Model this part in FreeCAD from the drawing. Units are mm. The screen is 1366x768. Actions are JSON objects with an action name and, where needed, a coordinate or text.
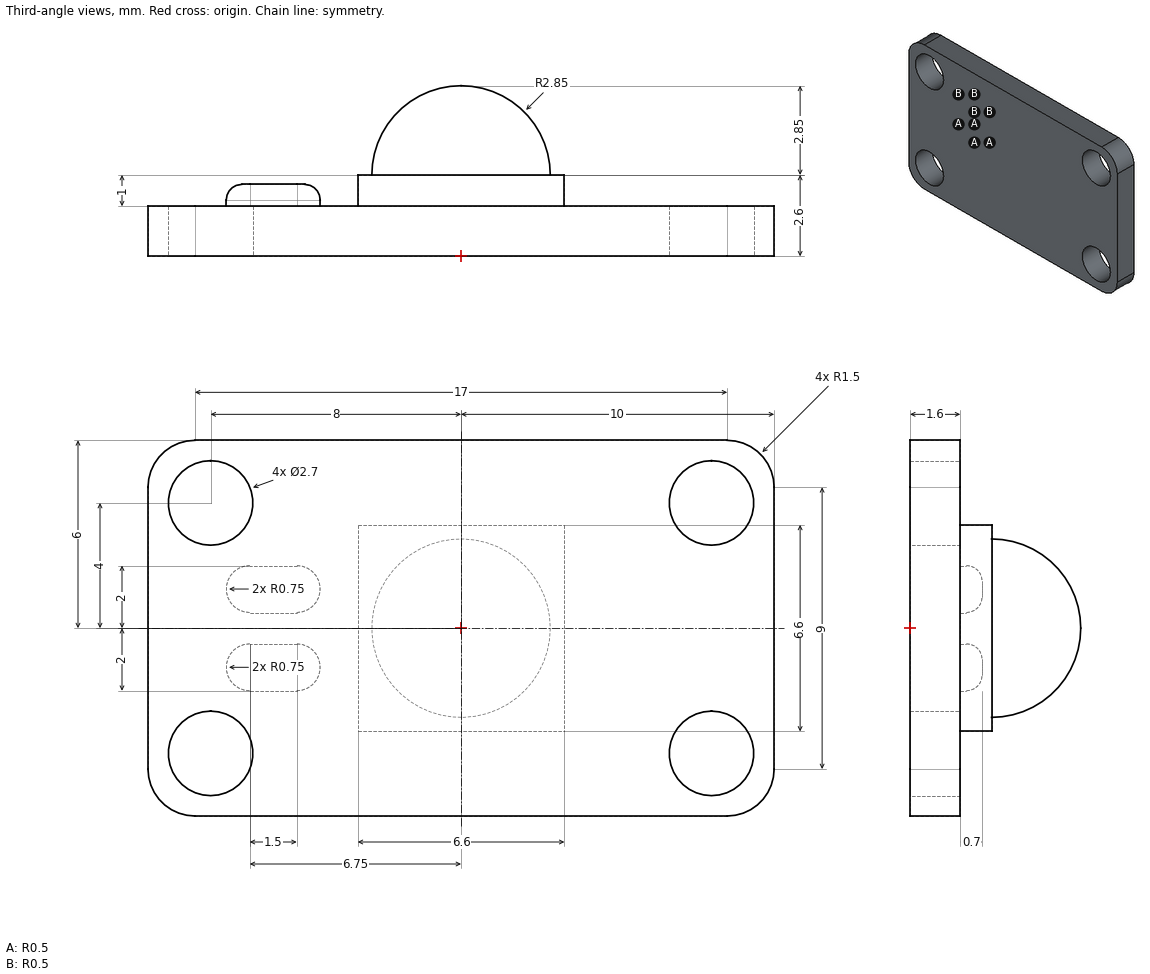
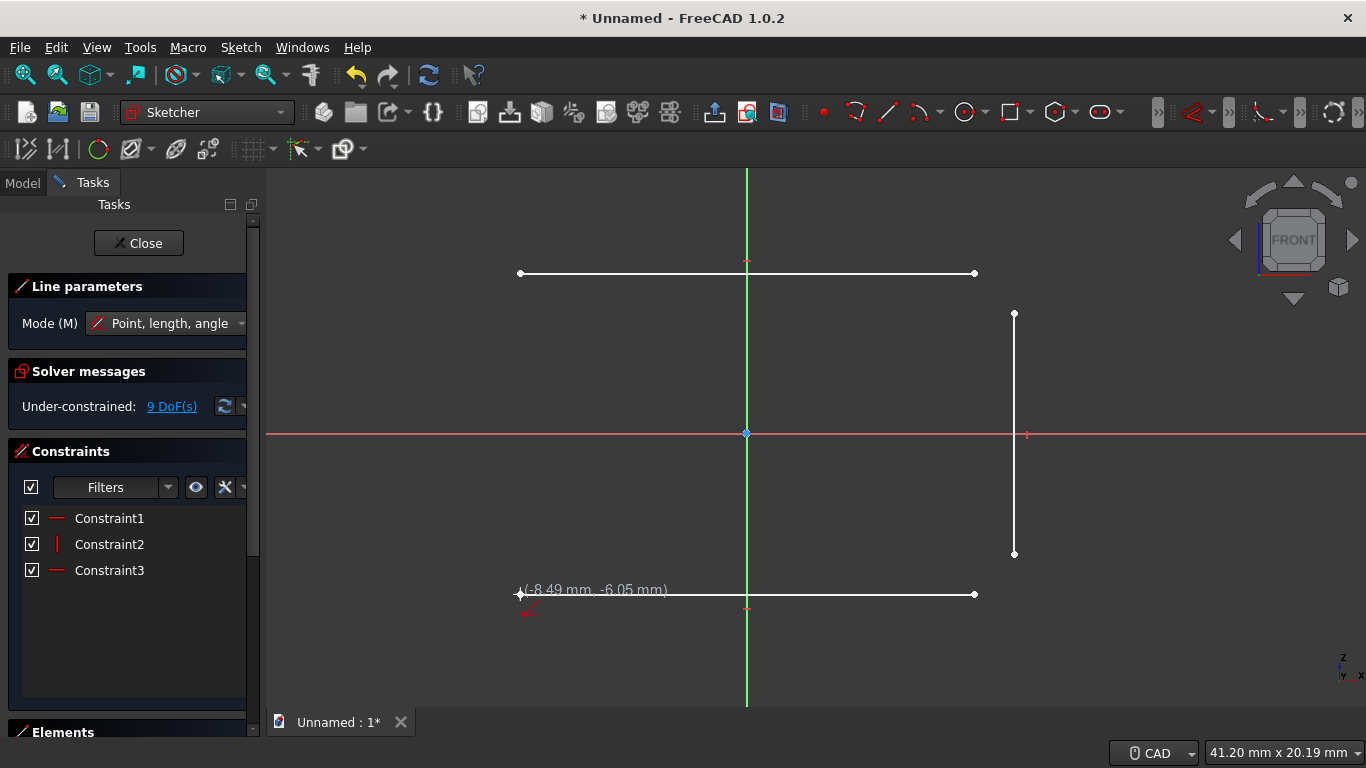
{"action": "left_click", "coordinate": [480, 554]}
{"action": "left_click", "coordinate": [480, 313]}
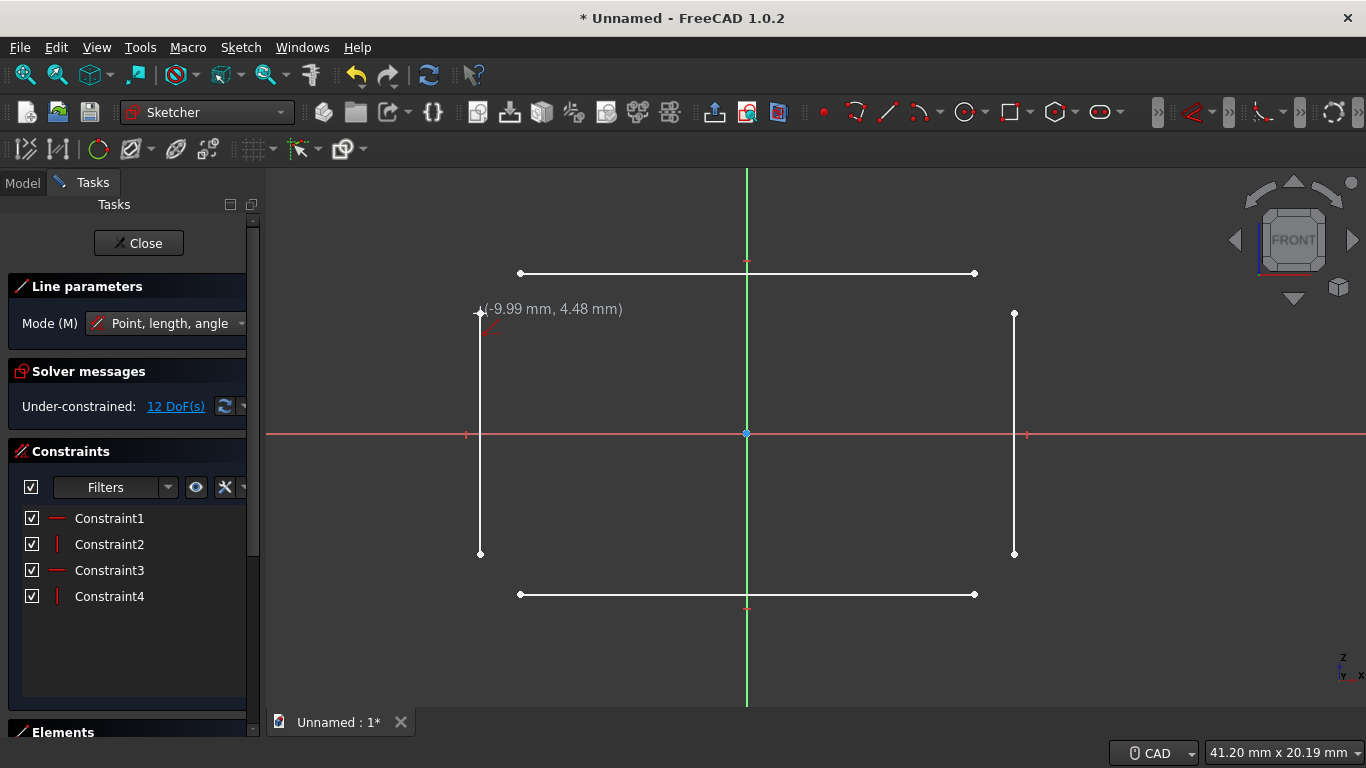
{"action": "left_click", "coordinate": [942, 112]}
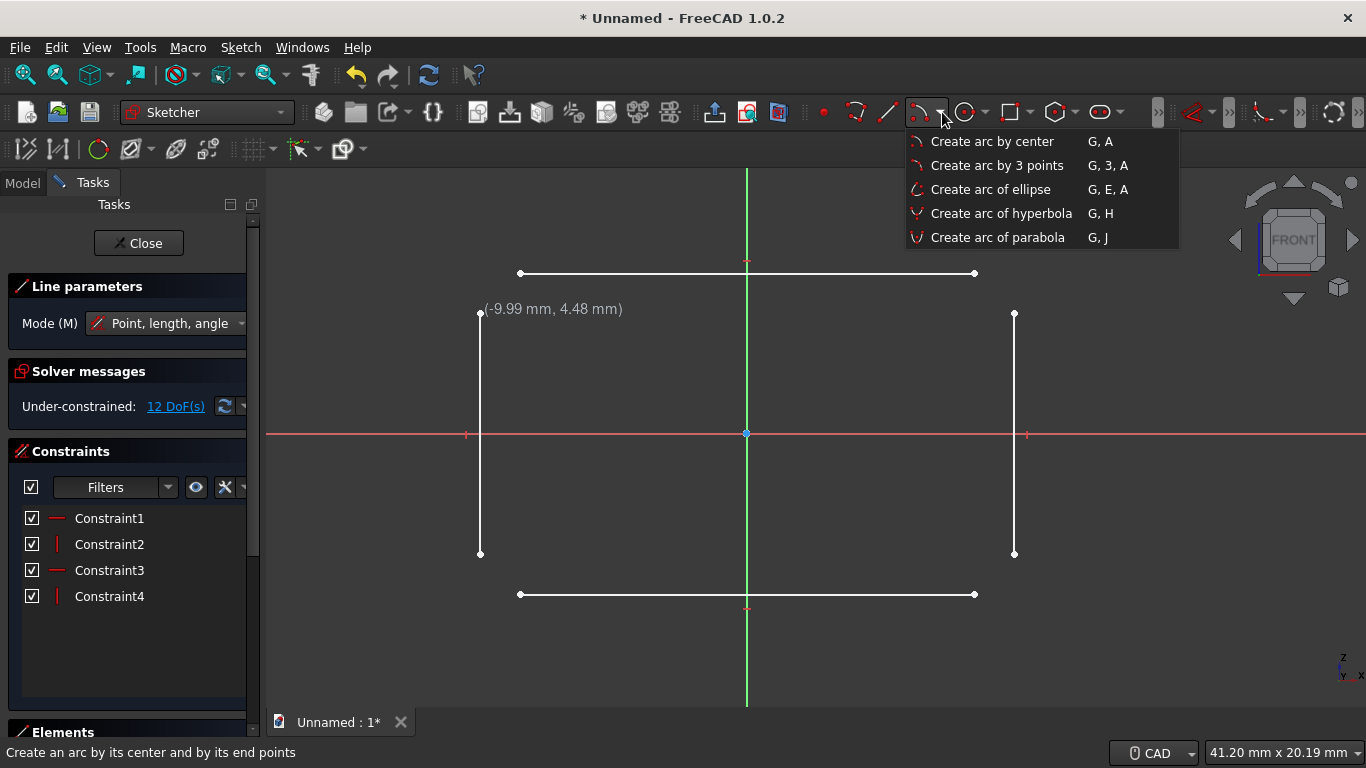
{"action": "left_click", "coordinate": [1042, 165]}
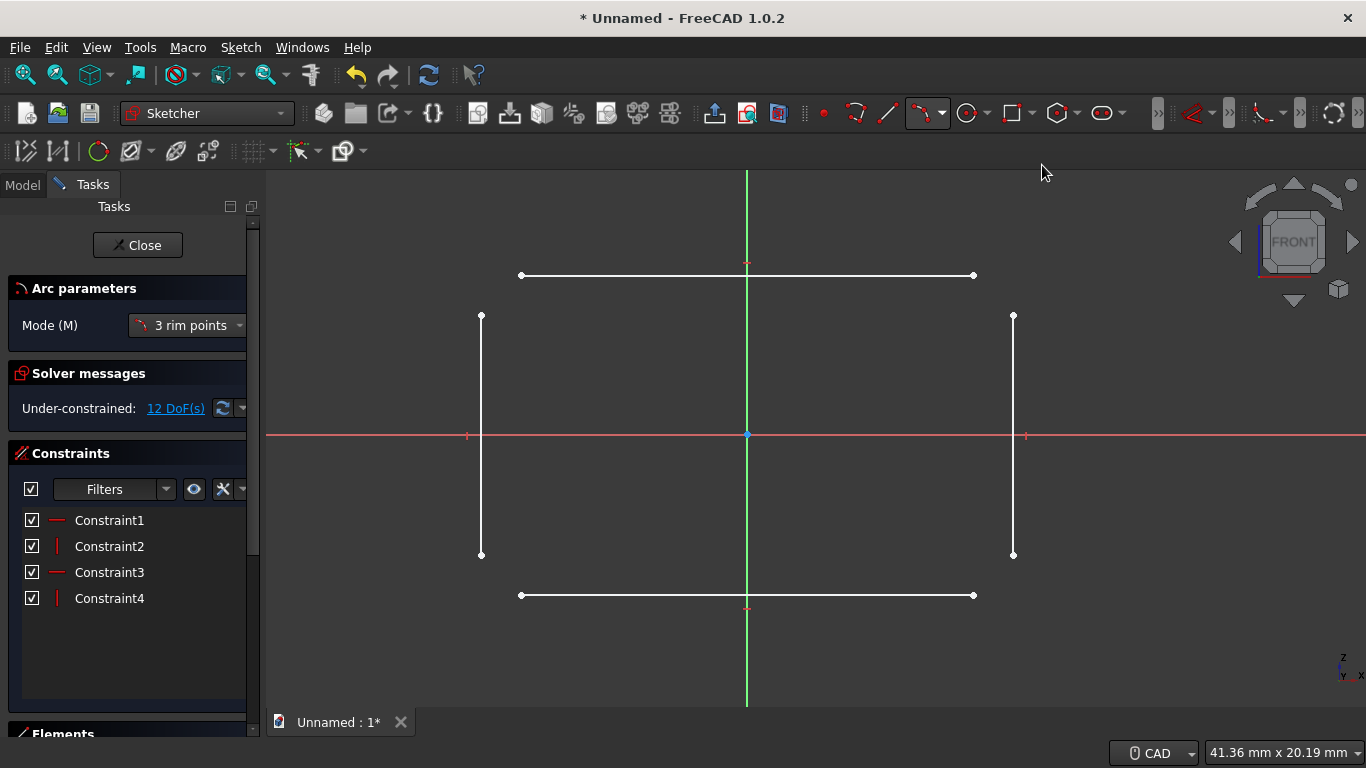
{"action": "left_click", "coordinate": [973, 276]}
{"action": "left_click", "coordinate": [1013, 315]}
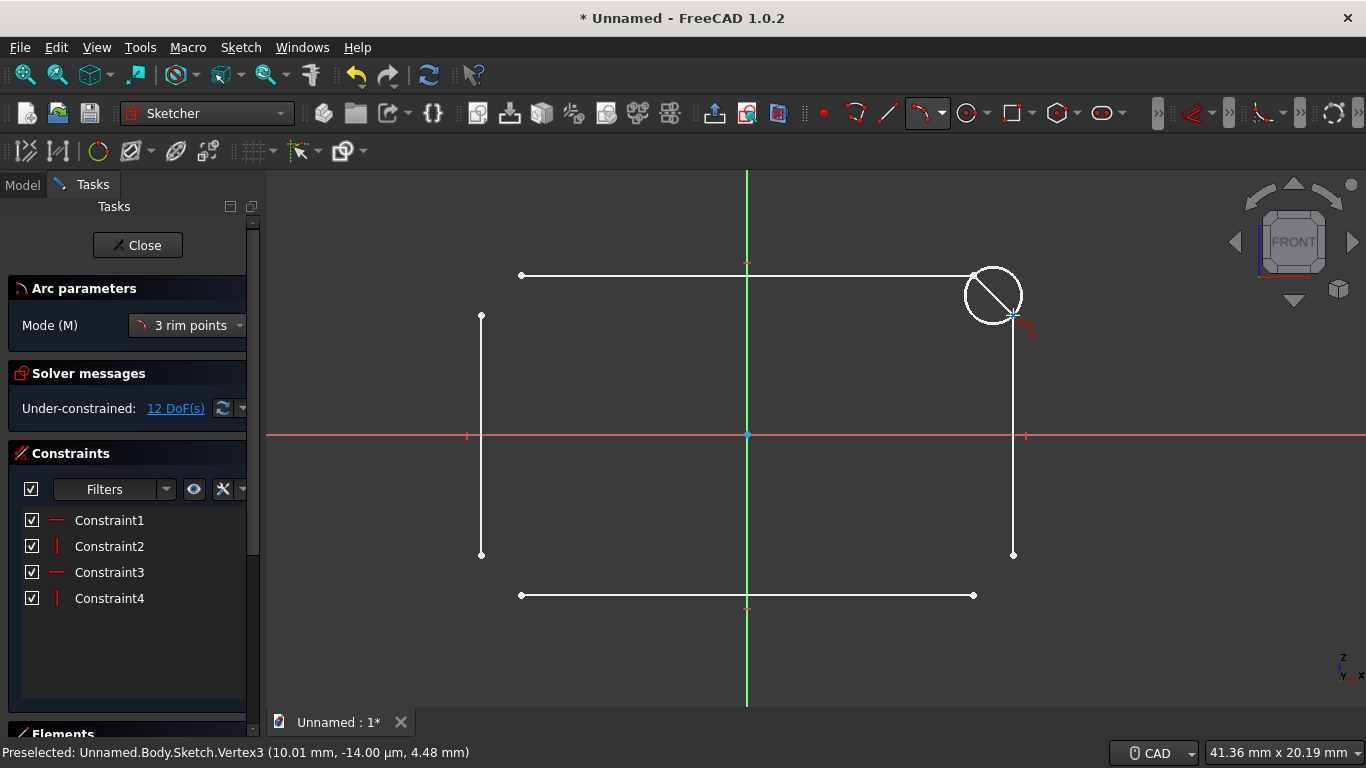
{"action": "scroll", "coordinate": [1001, 287], "scroll_direction": "up", "scroll_amount": 2}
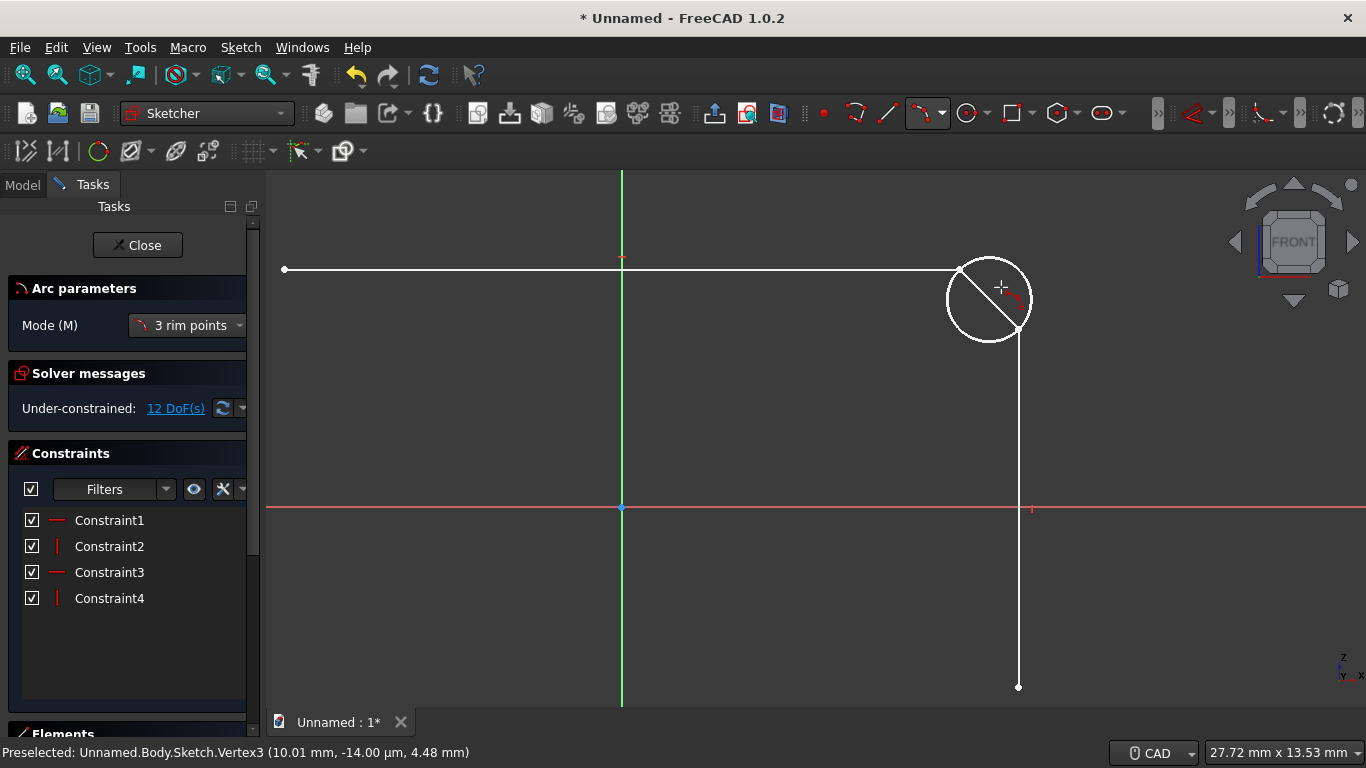
{"action": "left_click", "coordinate": [1001, 286]}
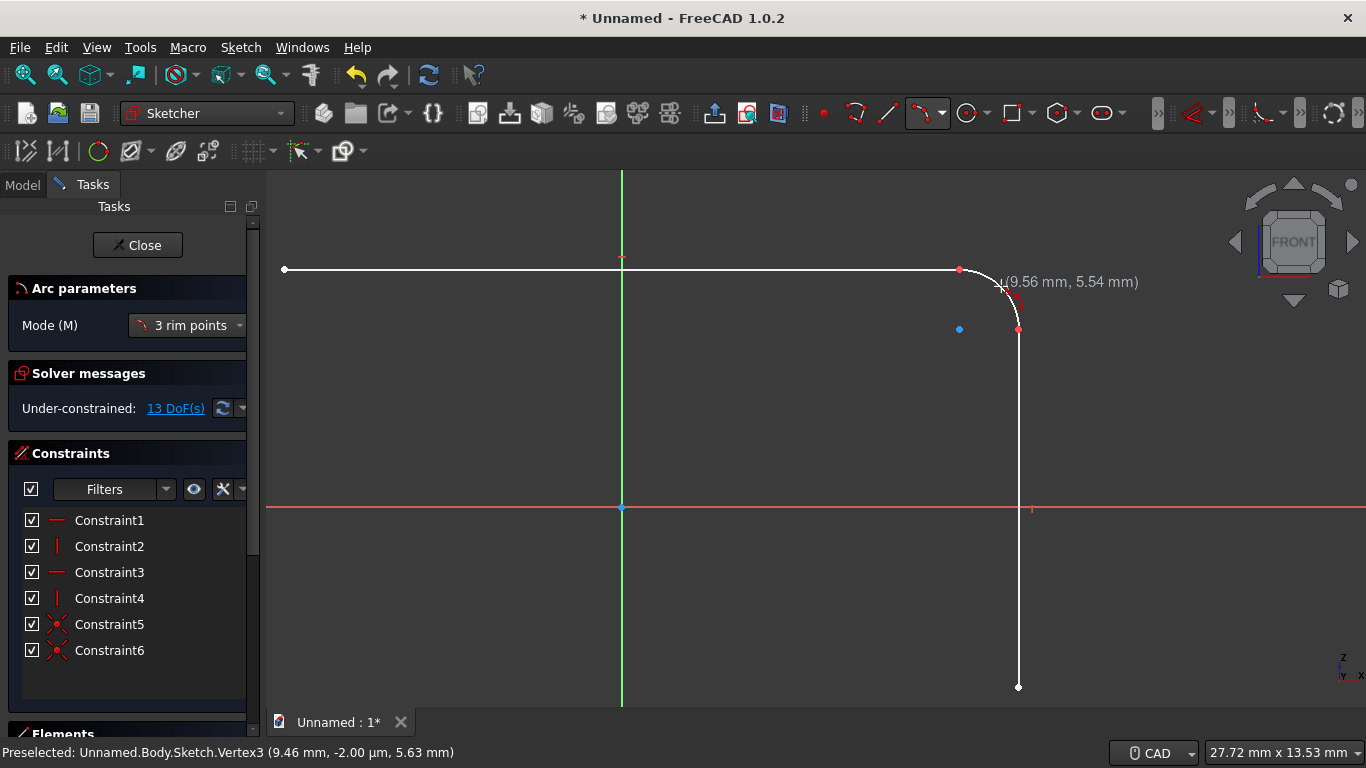
{"action": "scroll", "coordinate": [1003, 299], "scroll_direction": "down", "scroll_amount": 2}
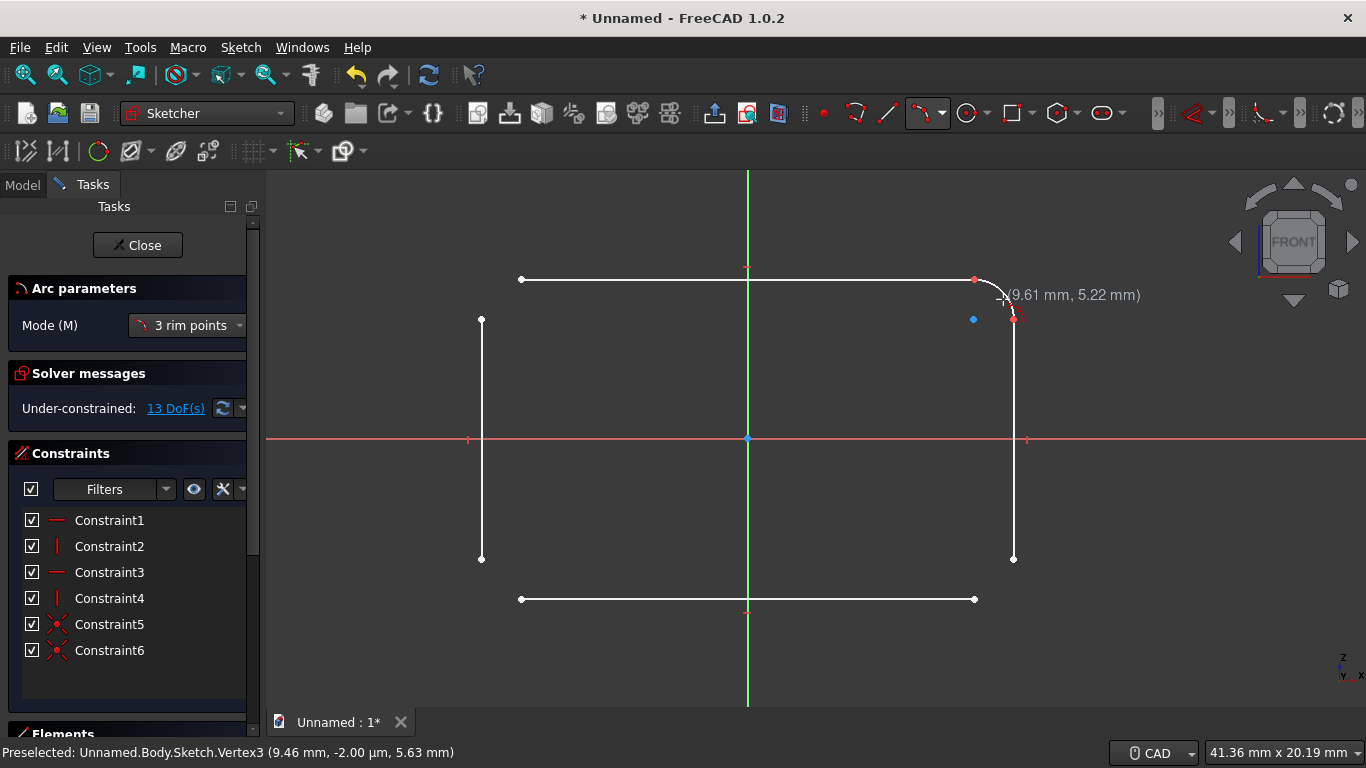
{"action": "left_click", "coordinate": [1014, 560]}
{"action": "left_click", "coordinate": [974, 599]}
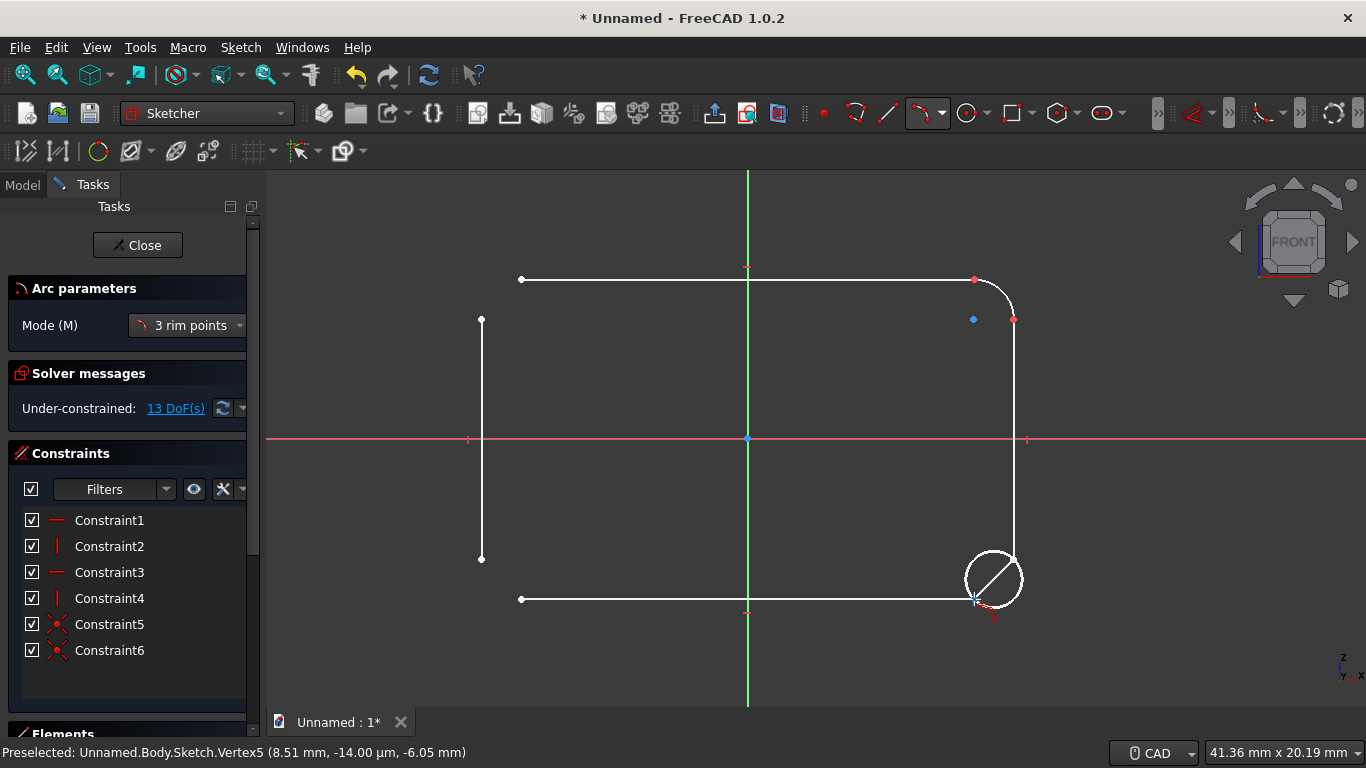
{"action": "scroll", "coordinate": [1002, 586], "scroll_direction": "up", "scroll_amount": 2}